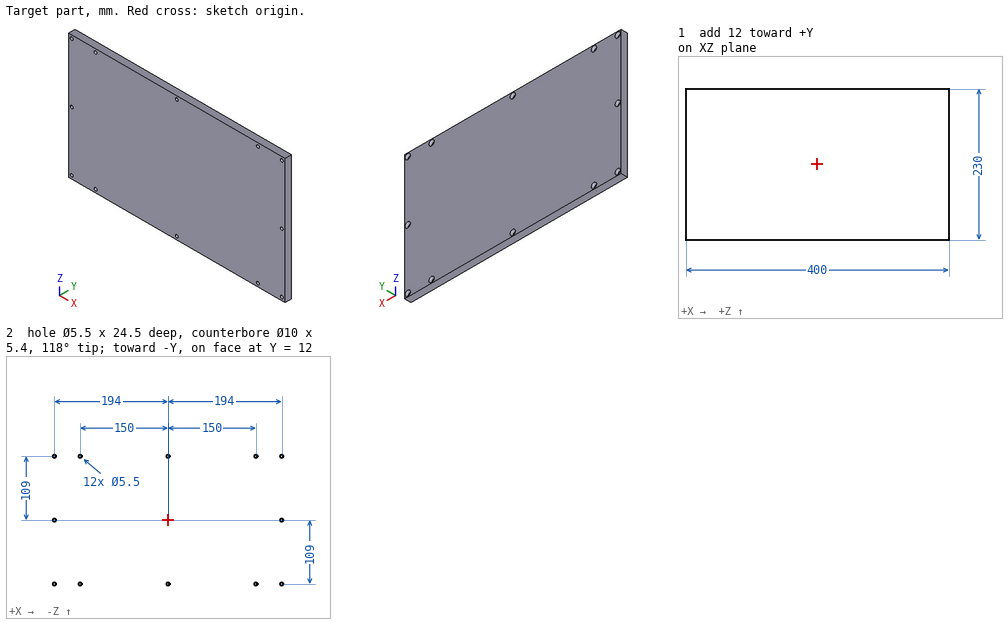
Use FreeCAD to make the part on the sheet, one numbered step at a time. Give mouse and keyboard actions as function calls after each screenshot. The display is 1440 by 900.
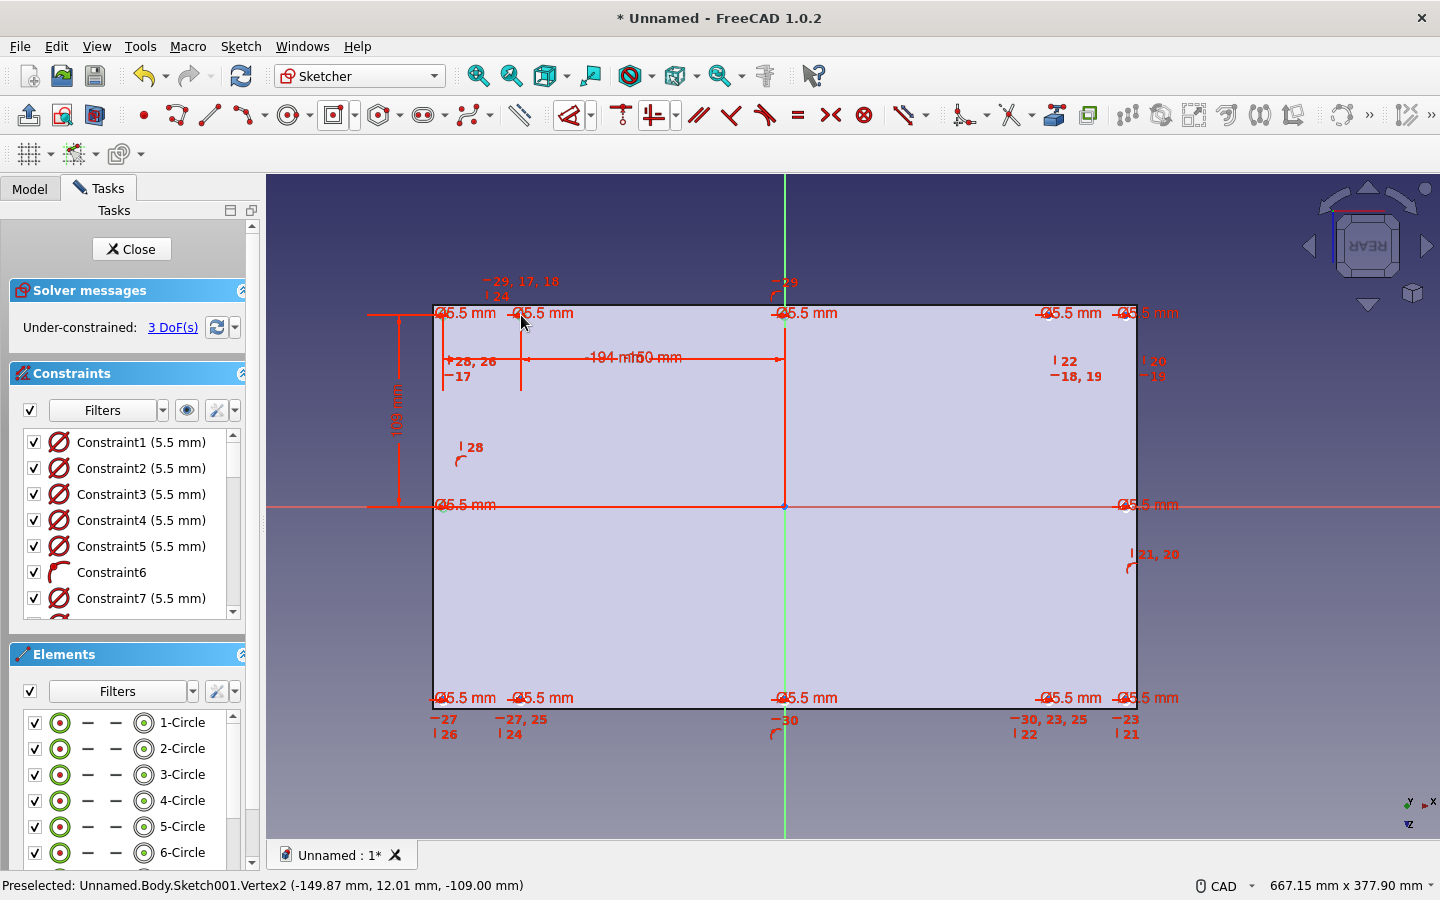
click(1049, 315)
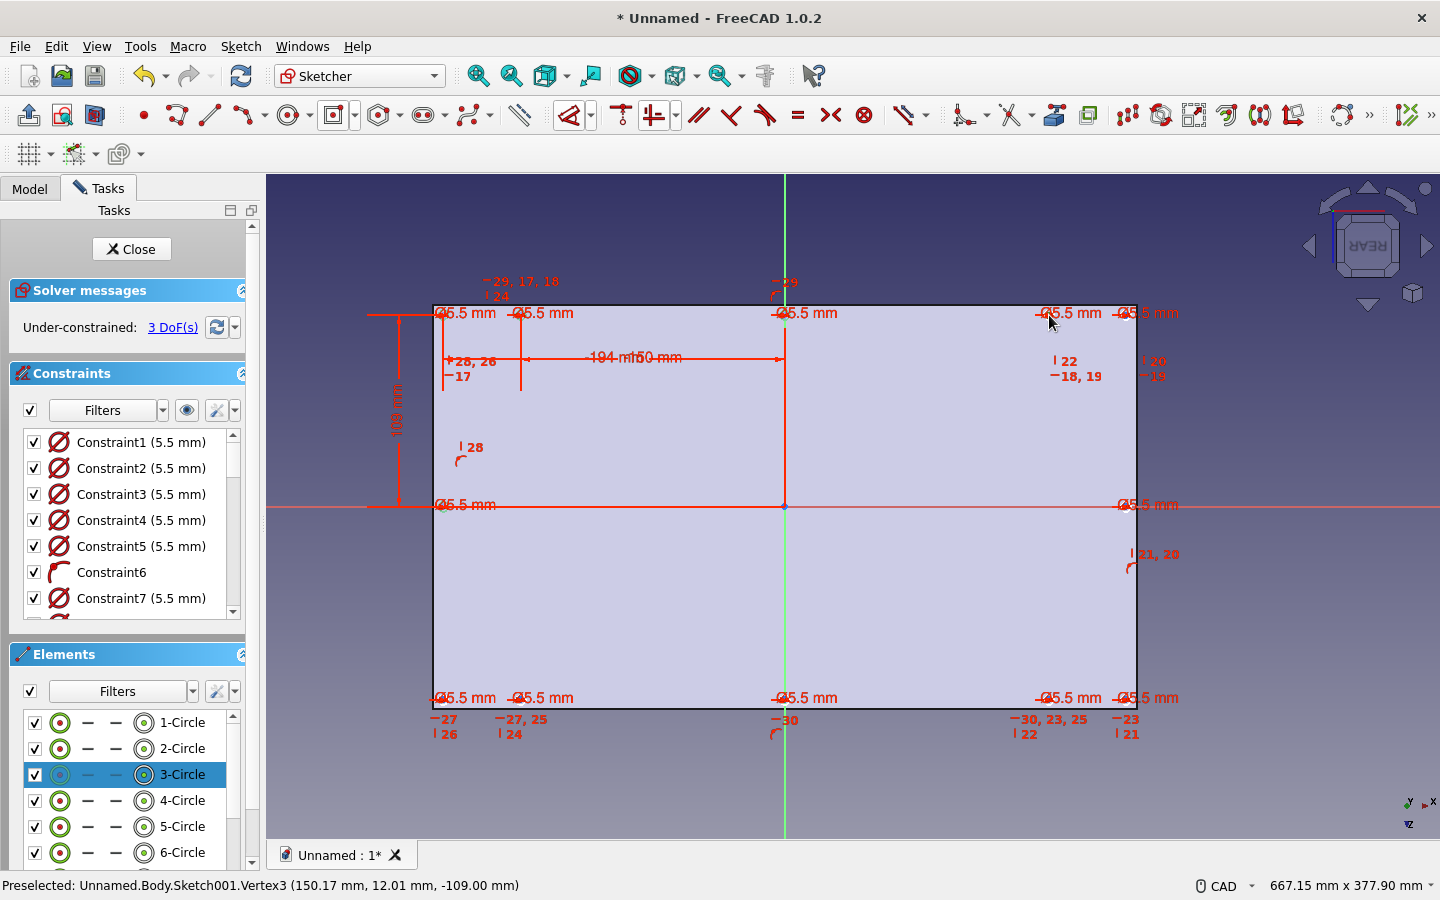
click(590, 116)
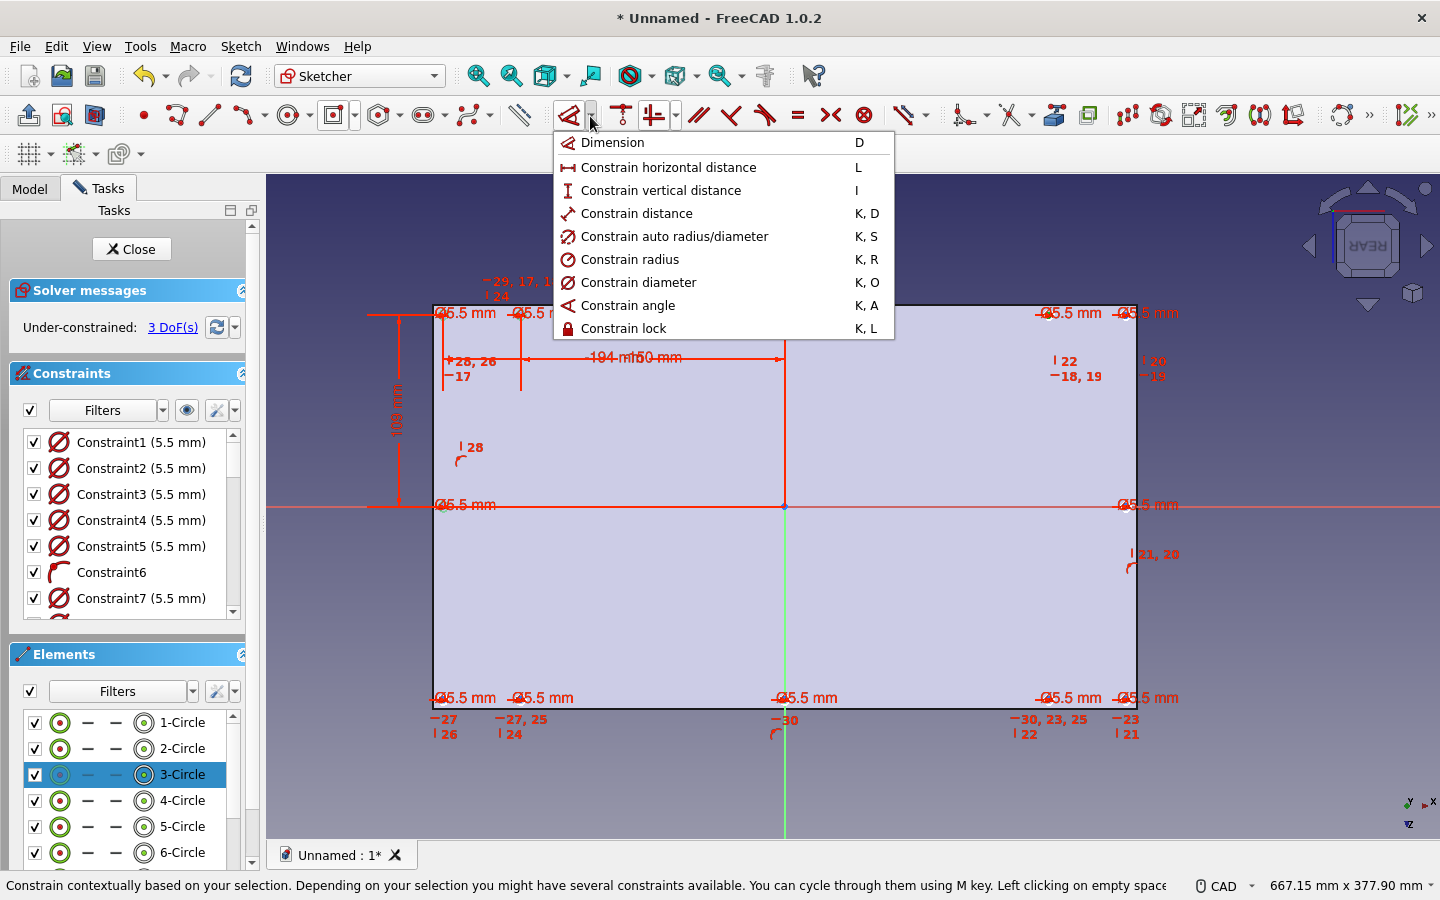
click(724, 168)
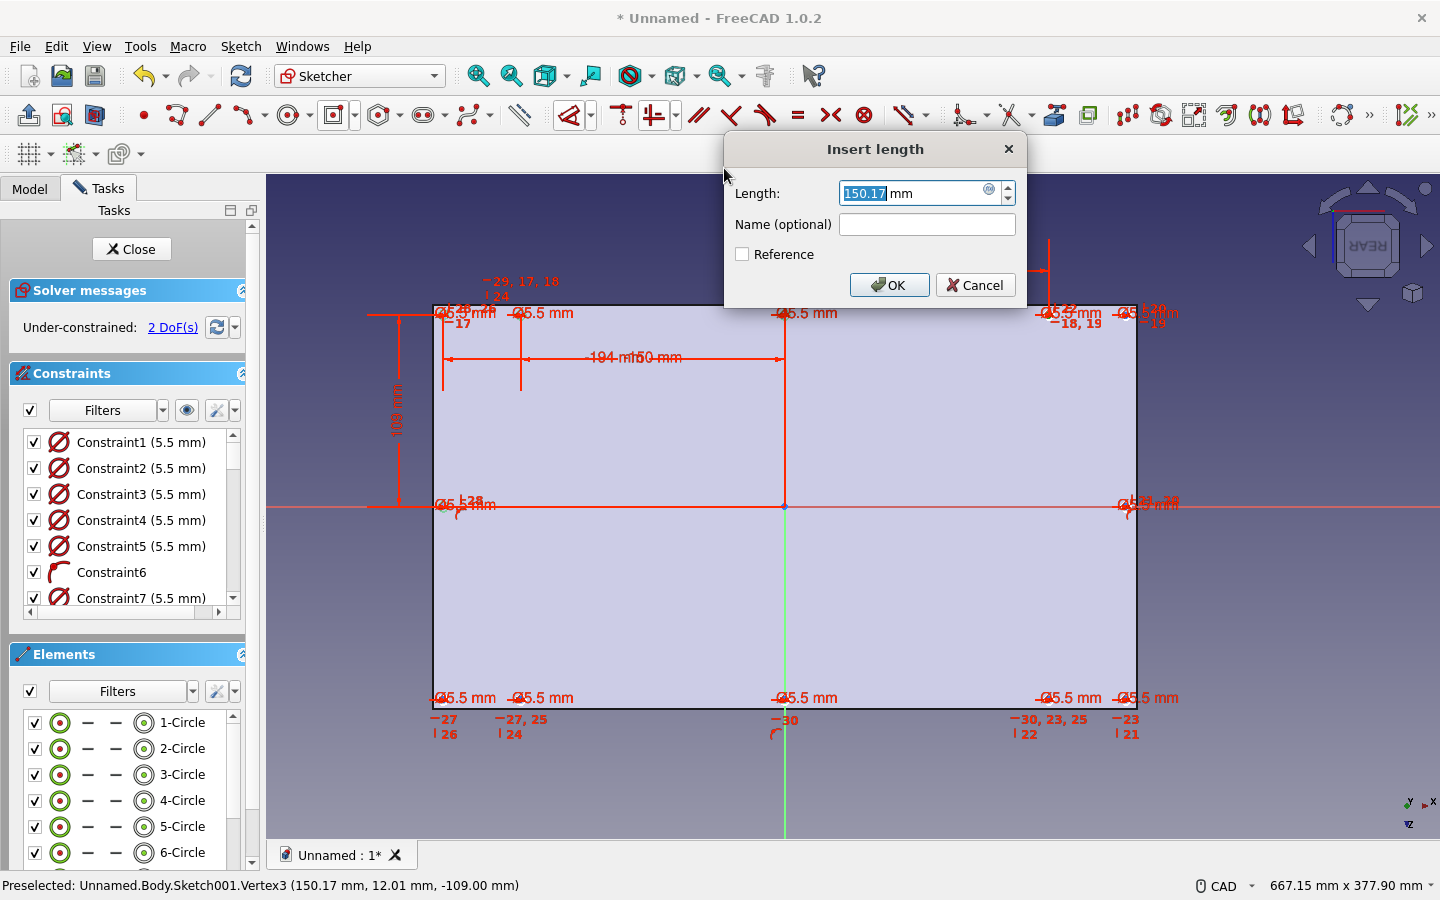
text(150)
key(Return)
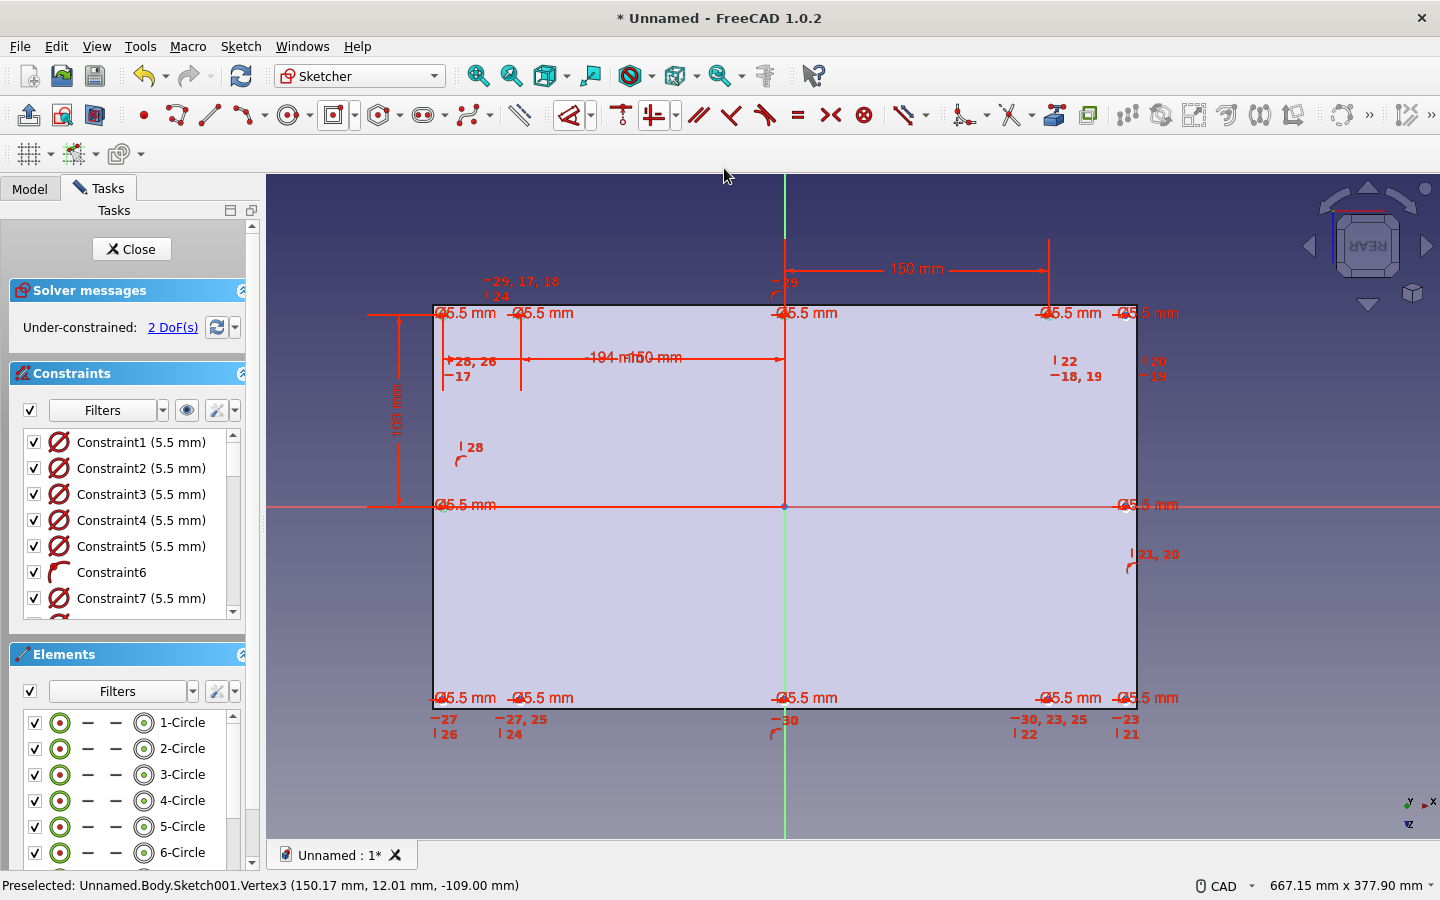
click(1126, 315)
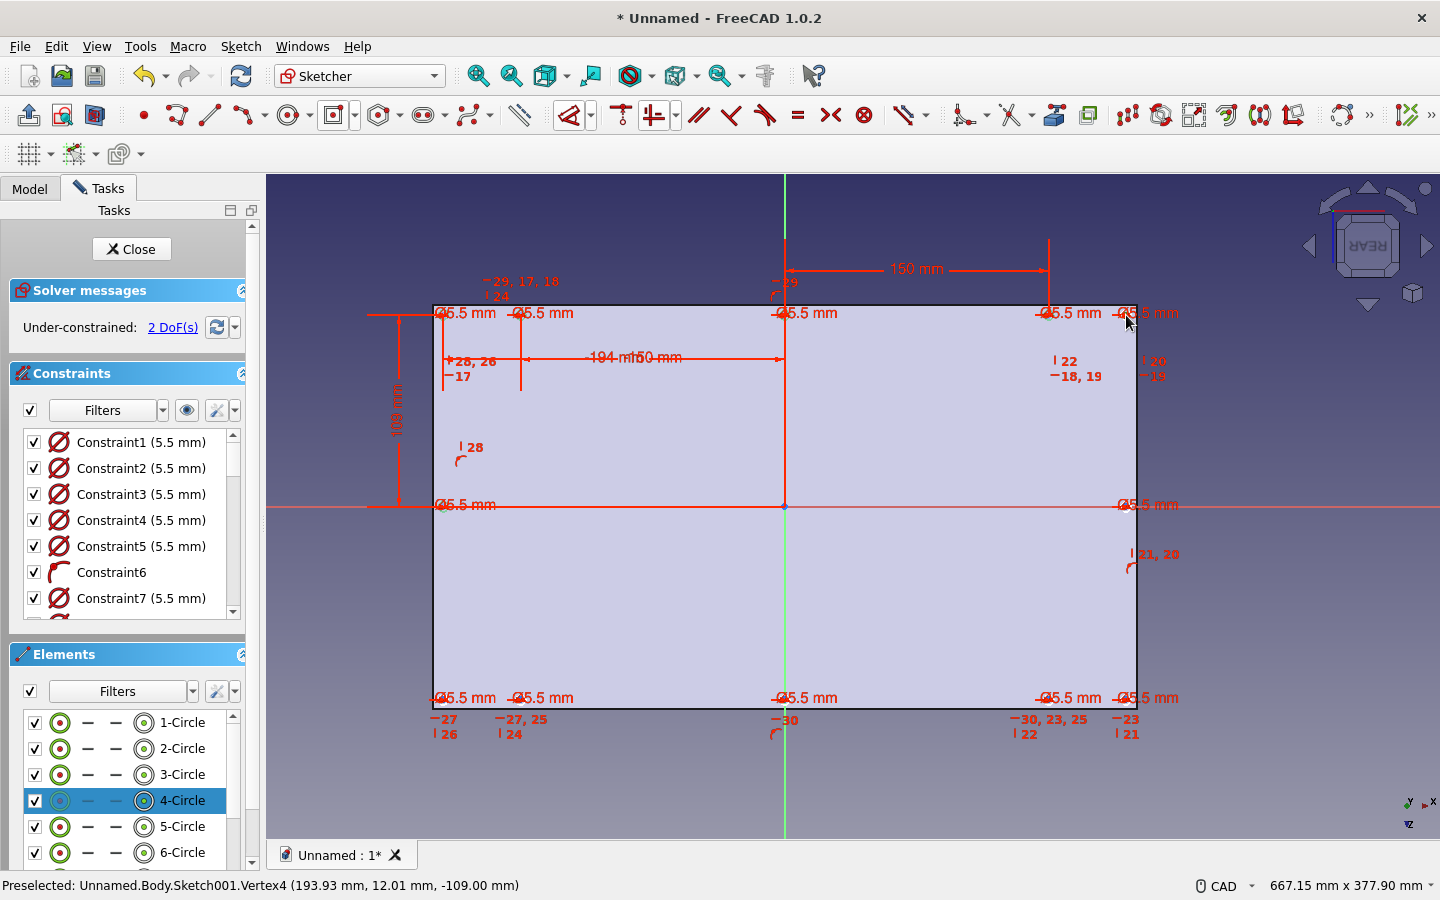
key(l)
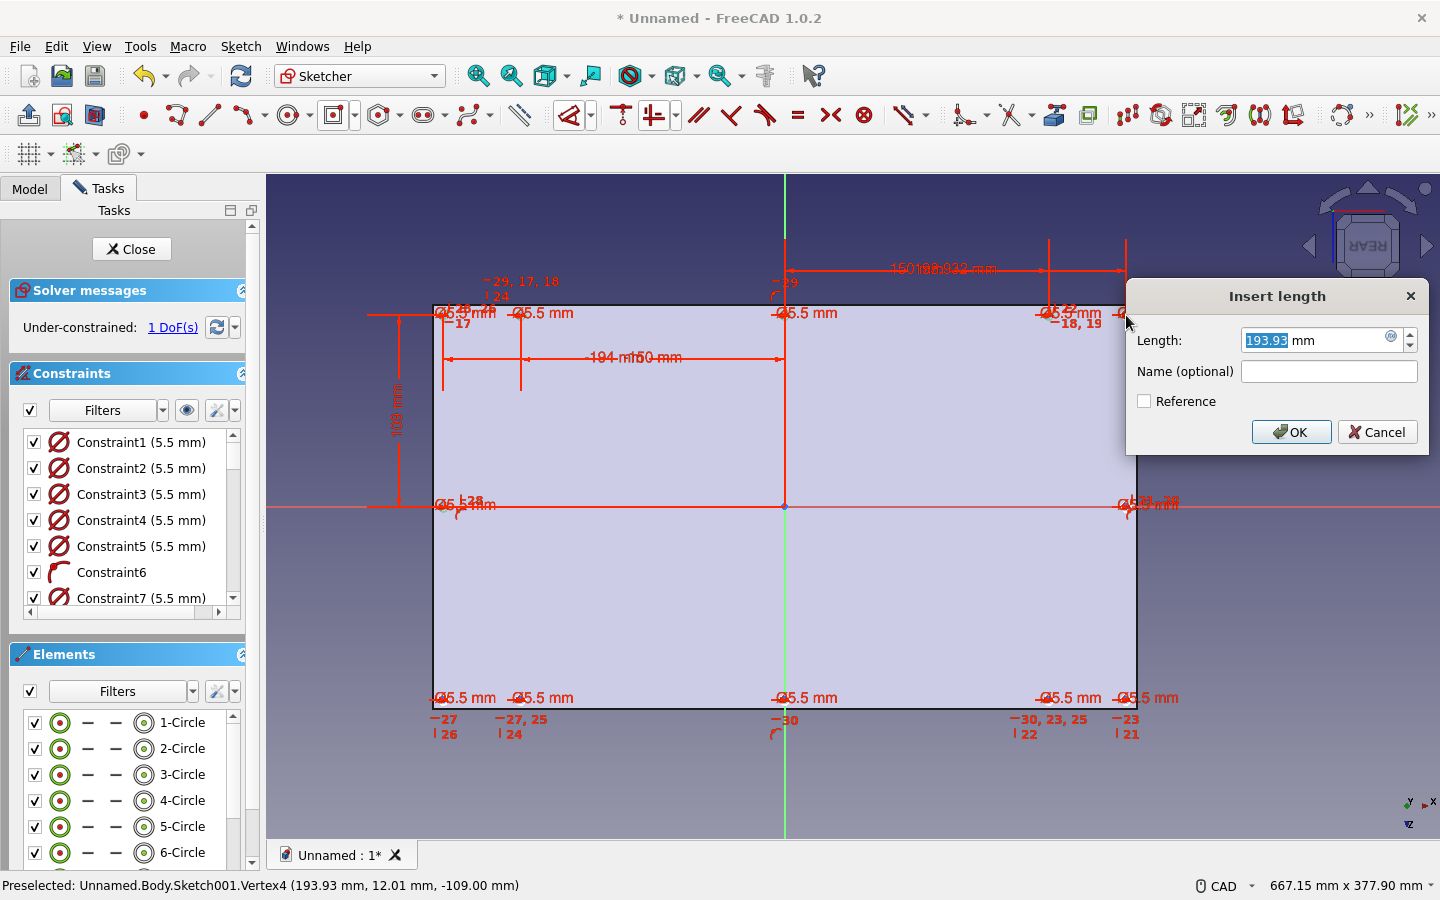
text(194)
key(Return)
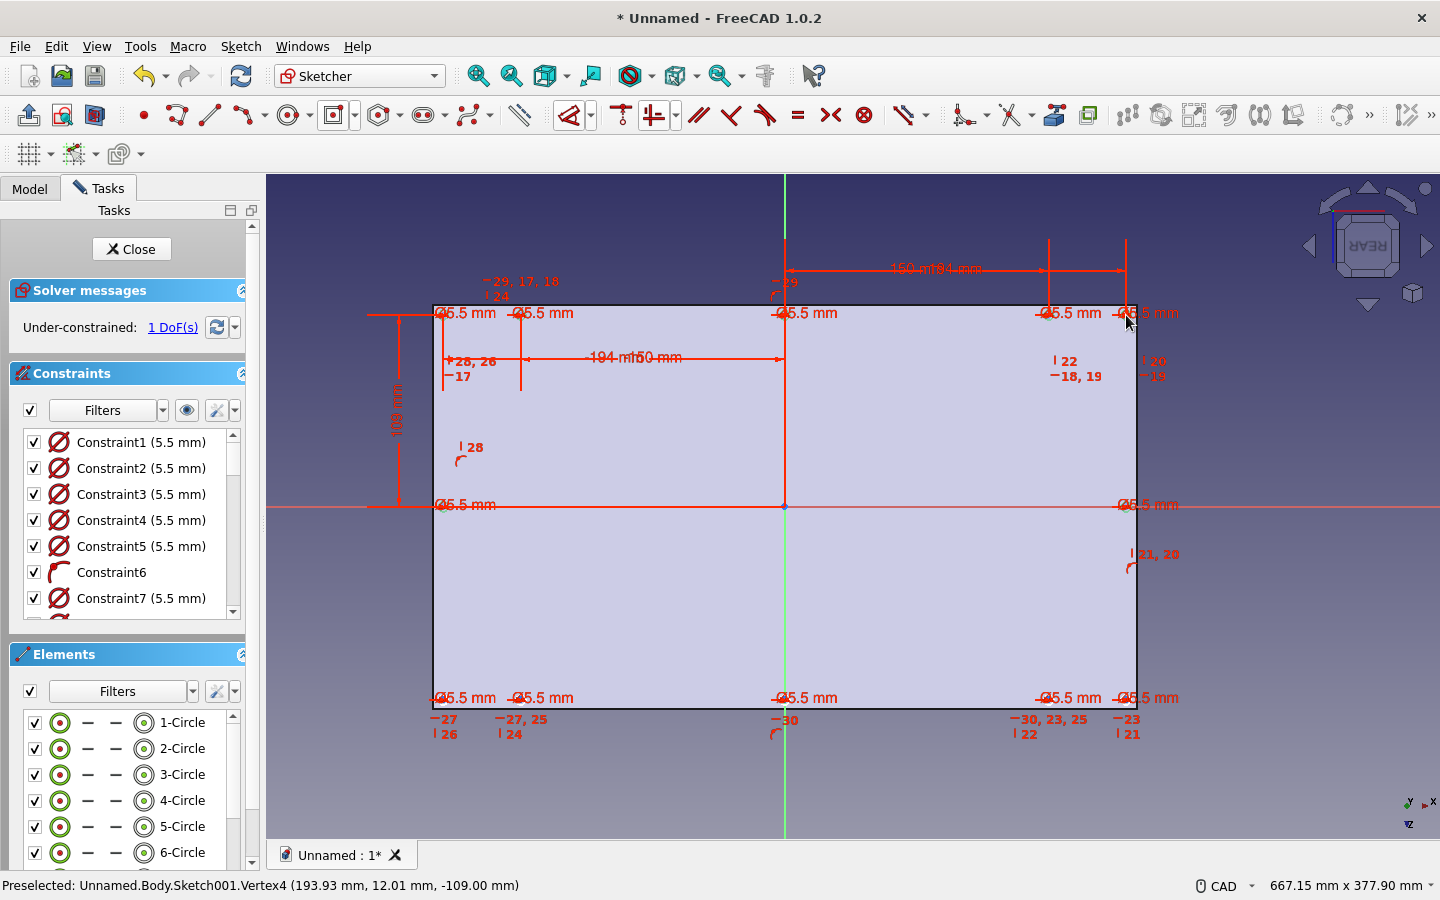
click(1126, 700)